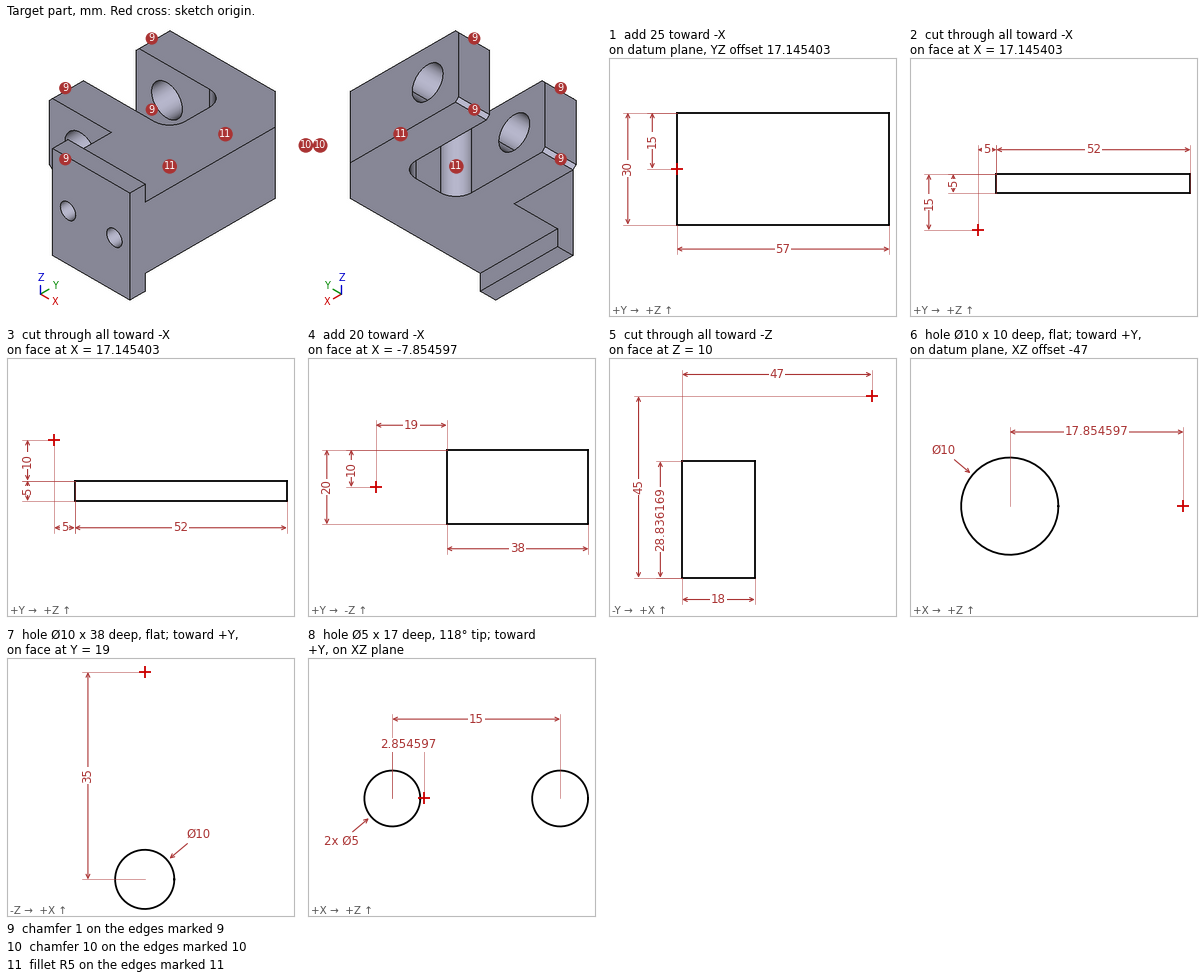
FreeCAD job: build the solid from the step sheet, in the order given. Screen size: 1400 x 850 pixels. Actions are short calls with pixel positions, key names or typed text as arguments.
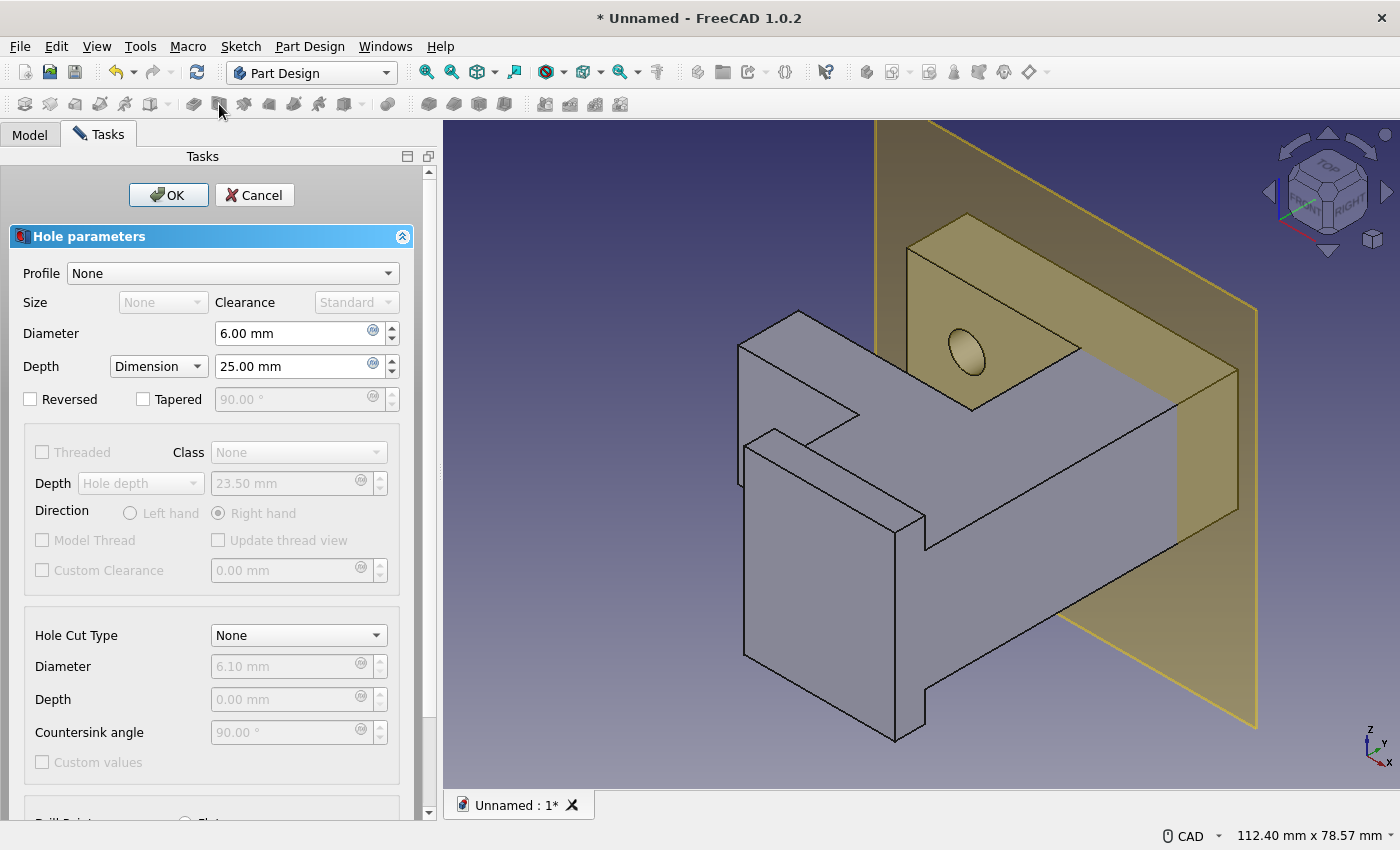
triple_click(300, 334)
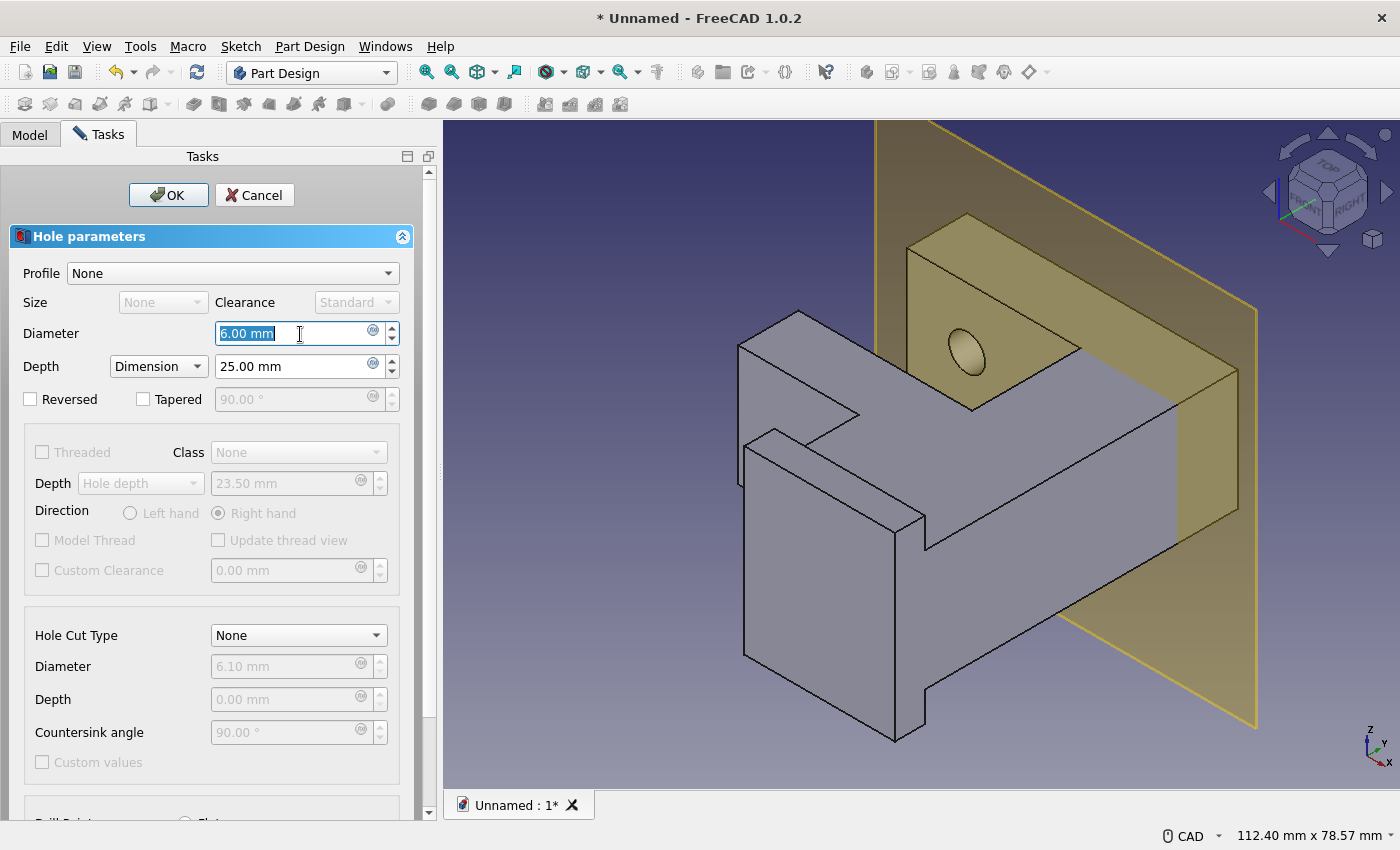
text(10)
key(Tab)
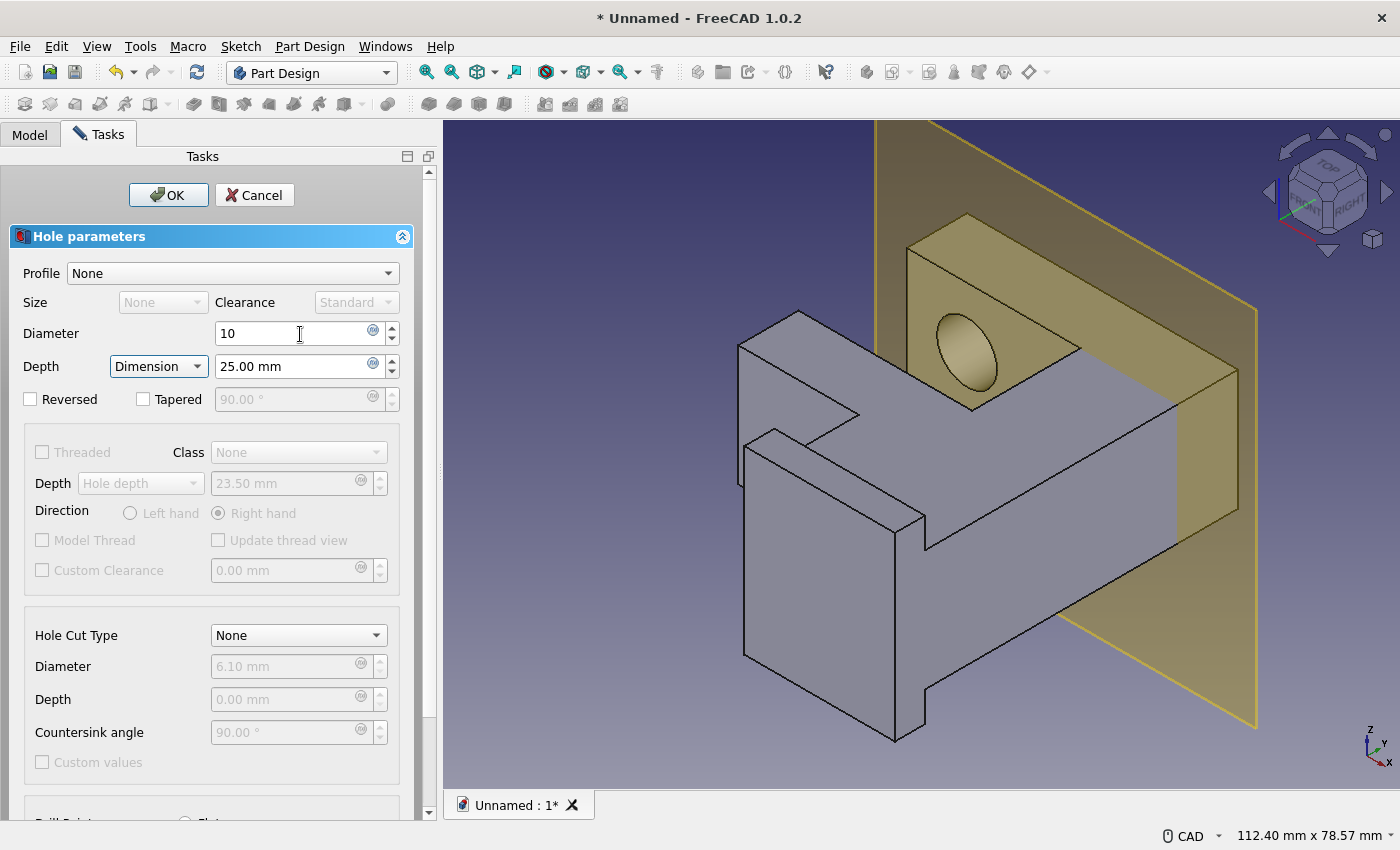
triple_click(300, 366)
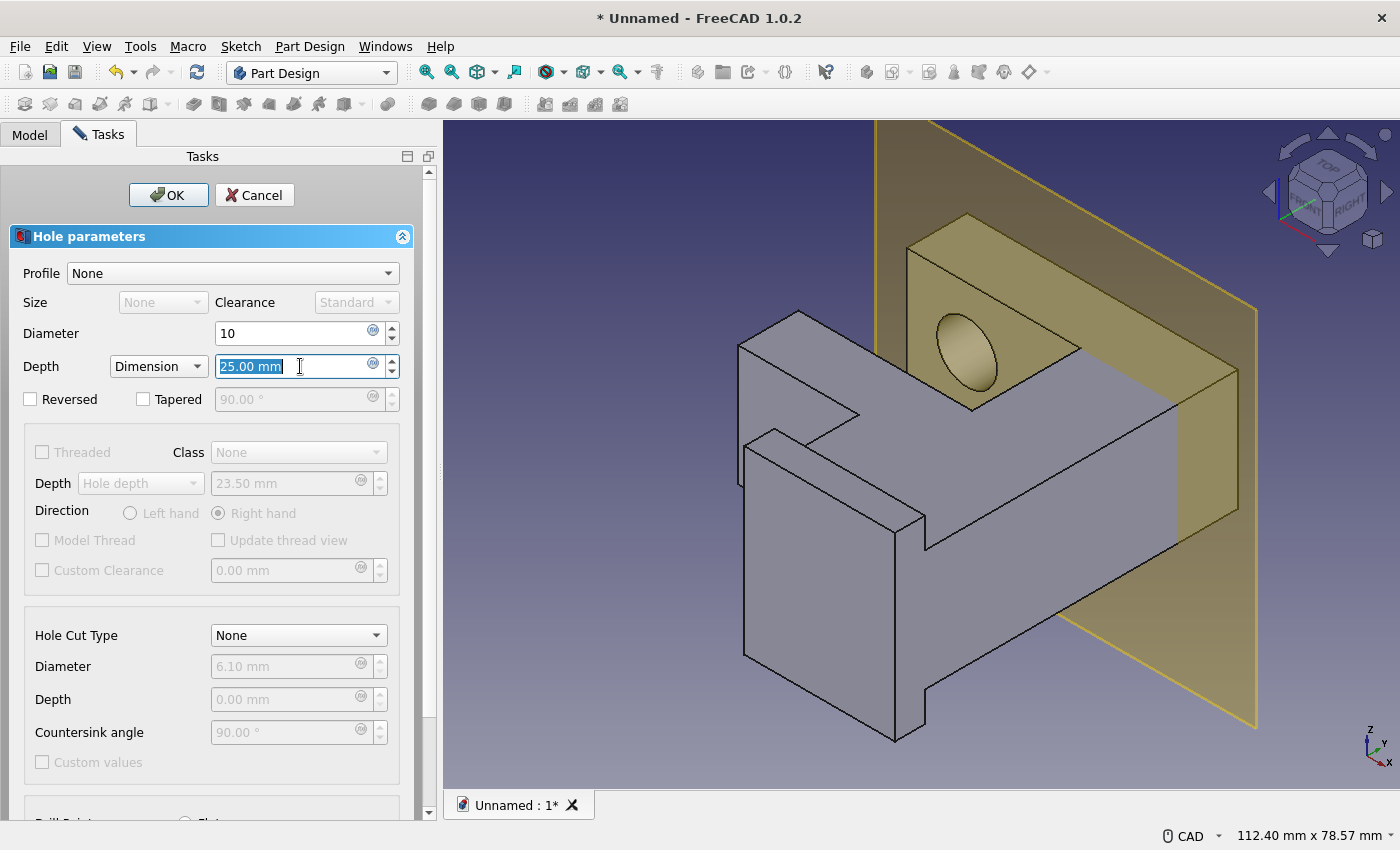
text(10)
key(Tab)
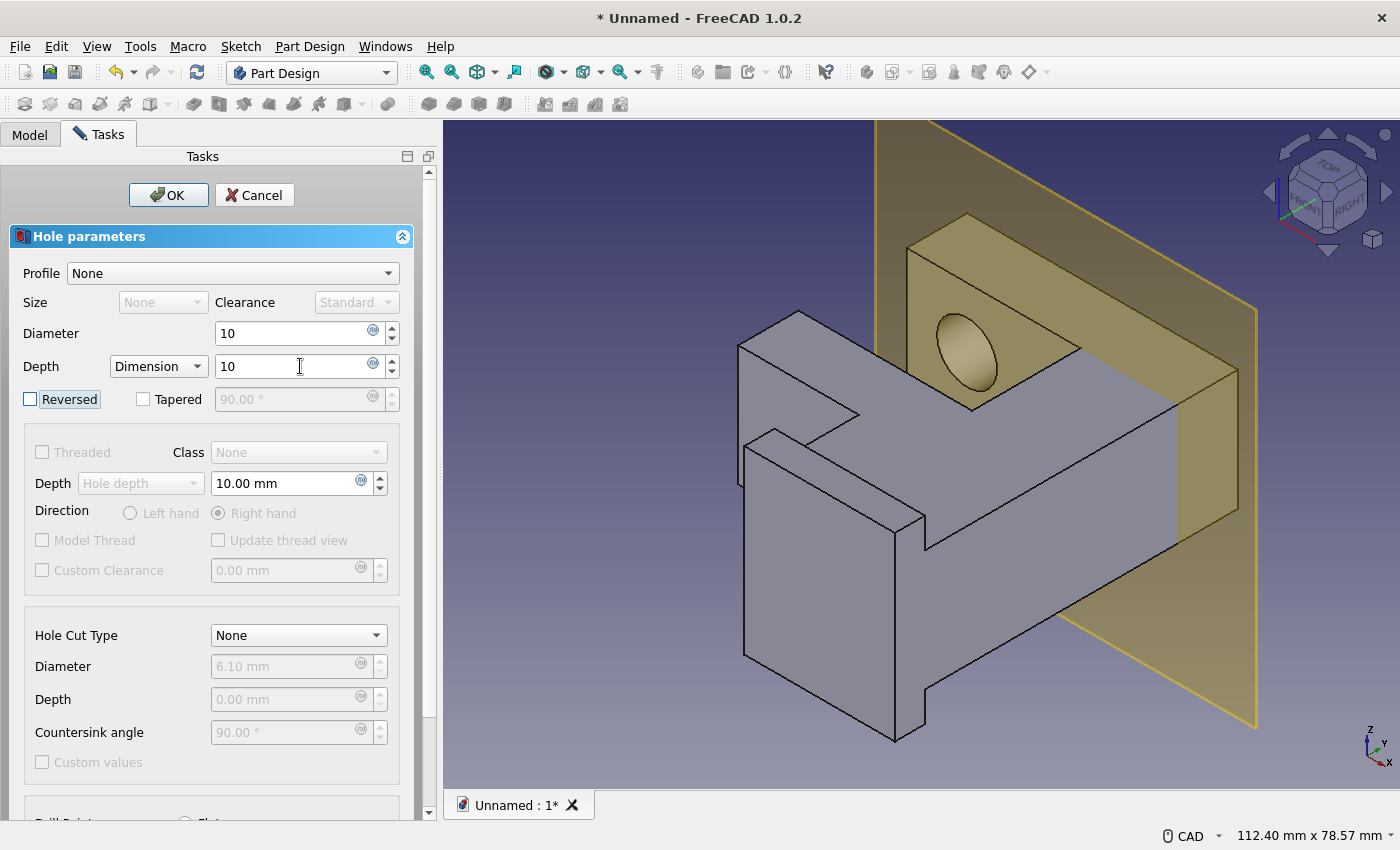
scroll(429, 493, down, 2)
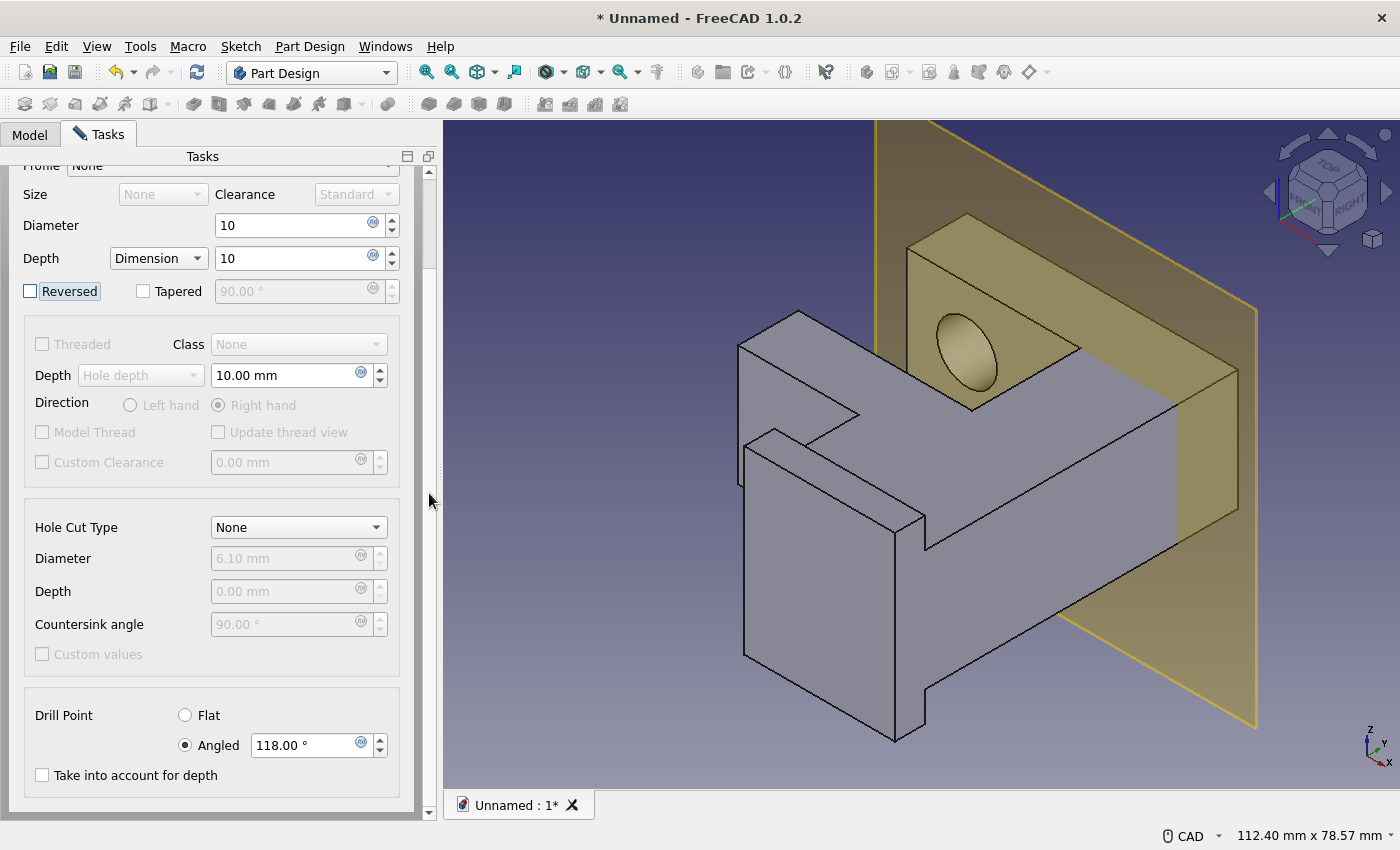
click(186, 713)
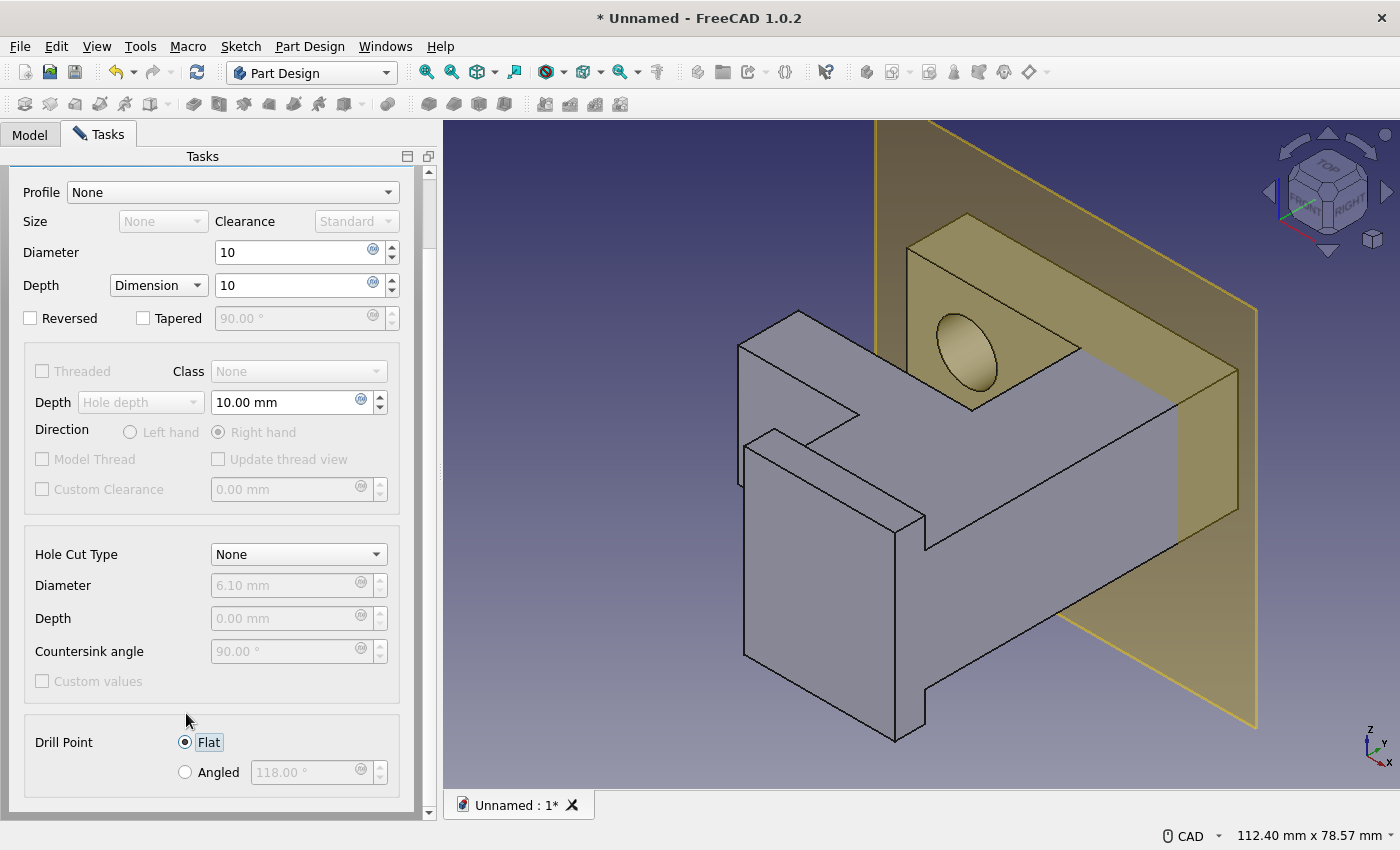
scroll(429, 493, up, 3)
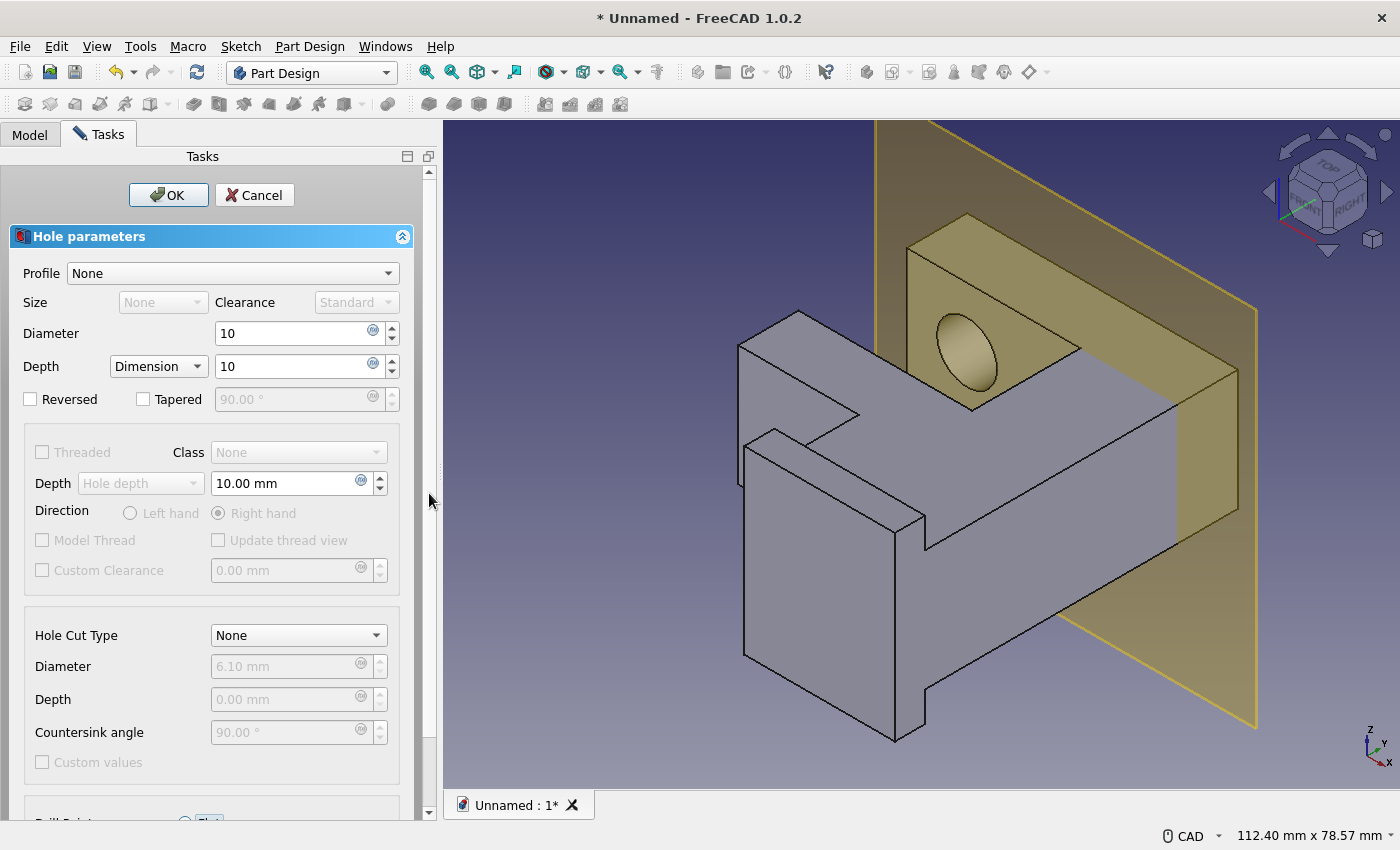
click(169, 195)